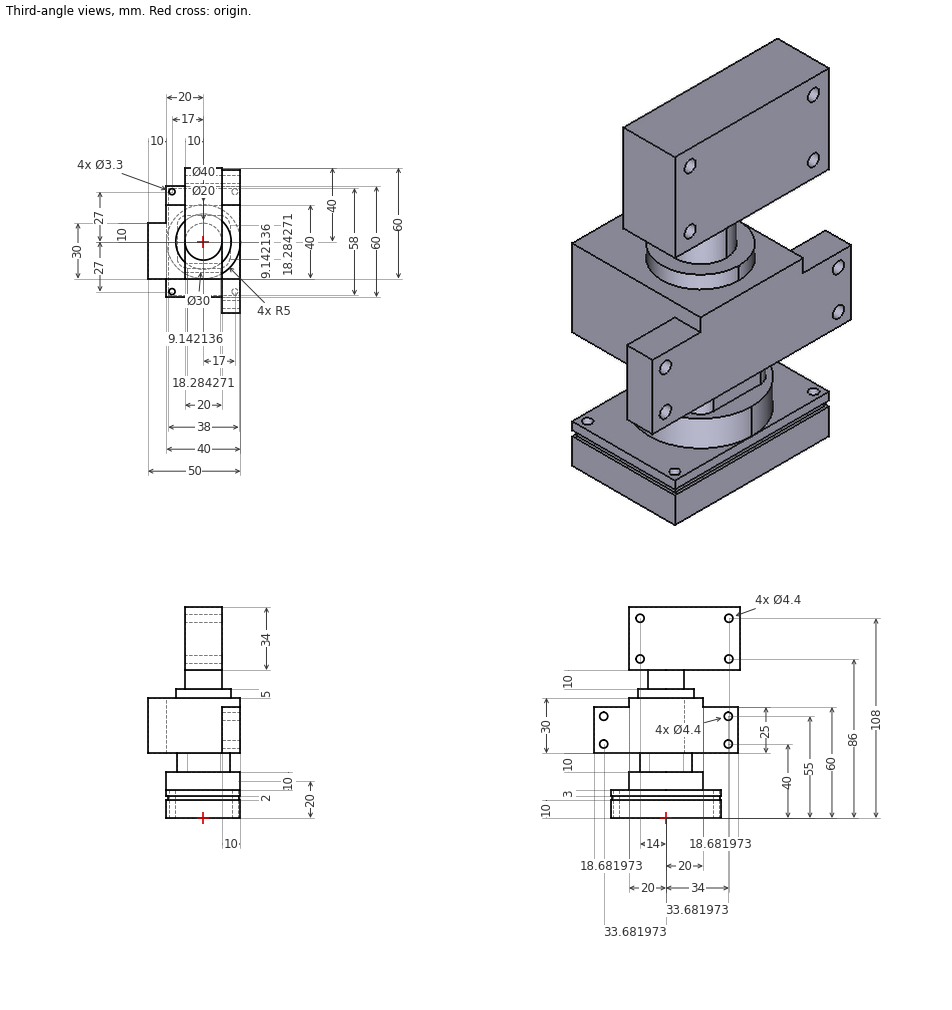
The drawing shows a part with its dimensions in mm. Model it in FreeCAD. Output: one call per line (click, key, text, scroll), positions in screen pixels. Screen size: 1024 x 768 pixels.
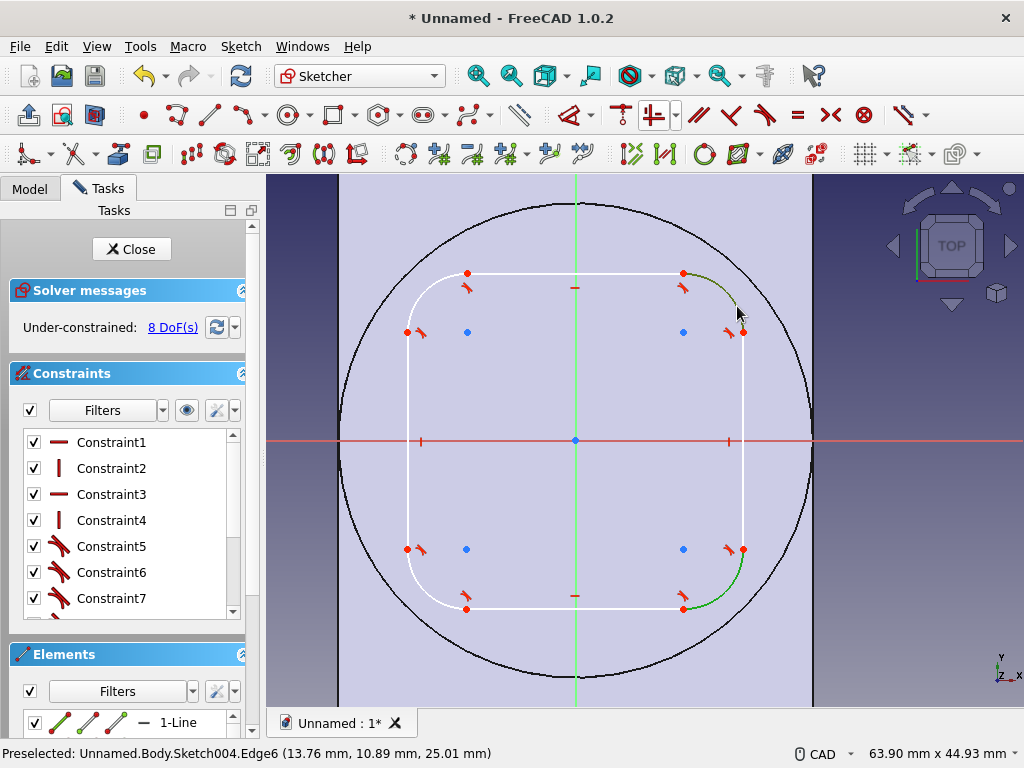
click(440, 280)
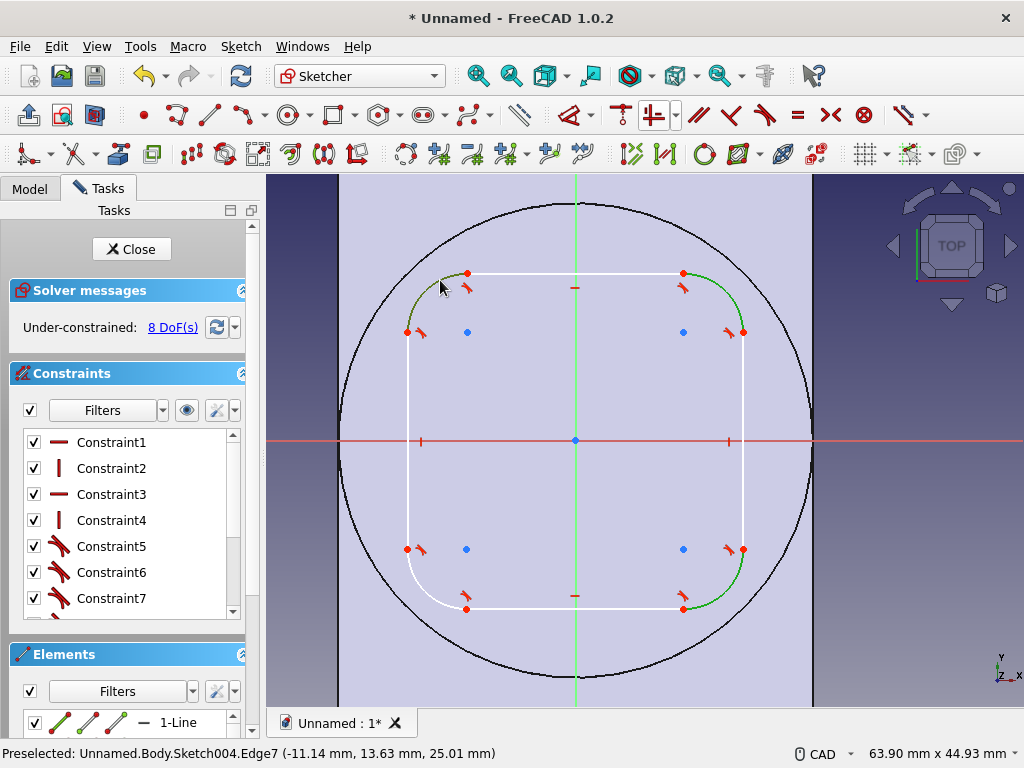
click(414, 577)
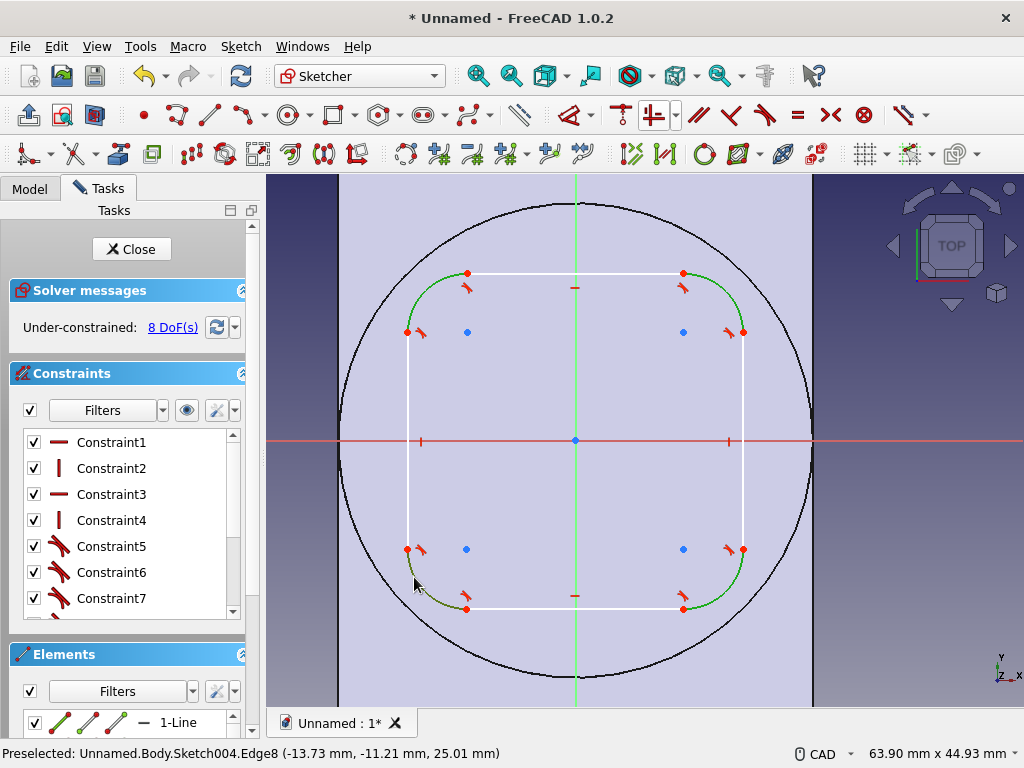
key(e)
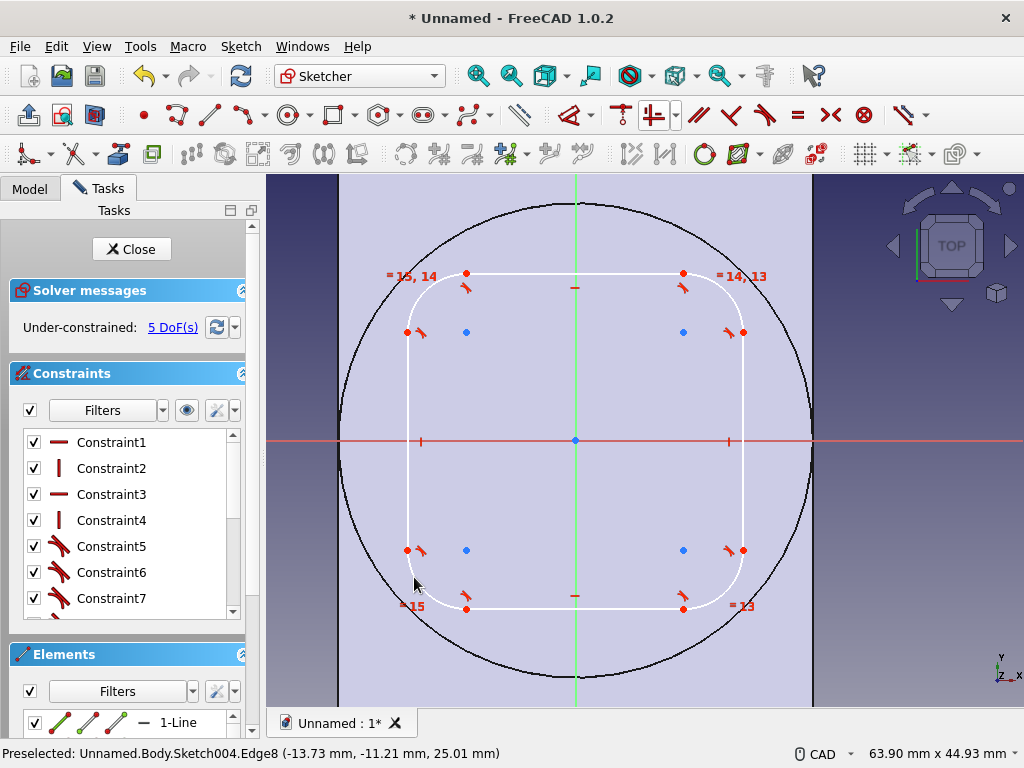
key(d)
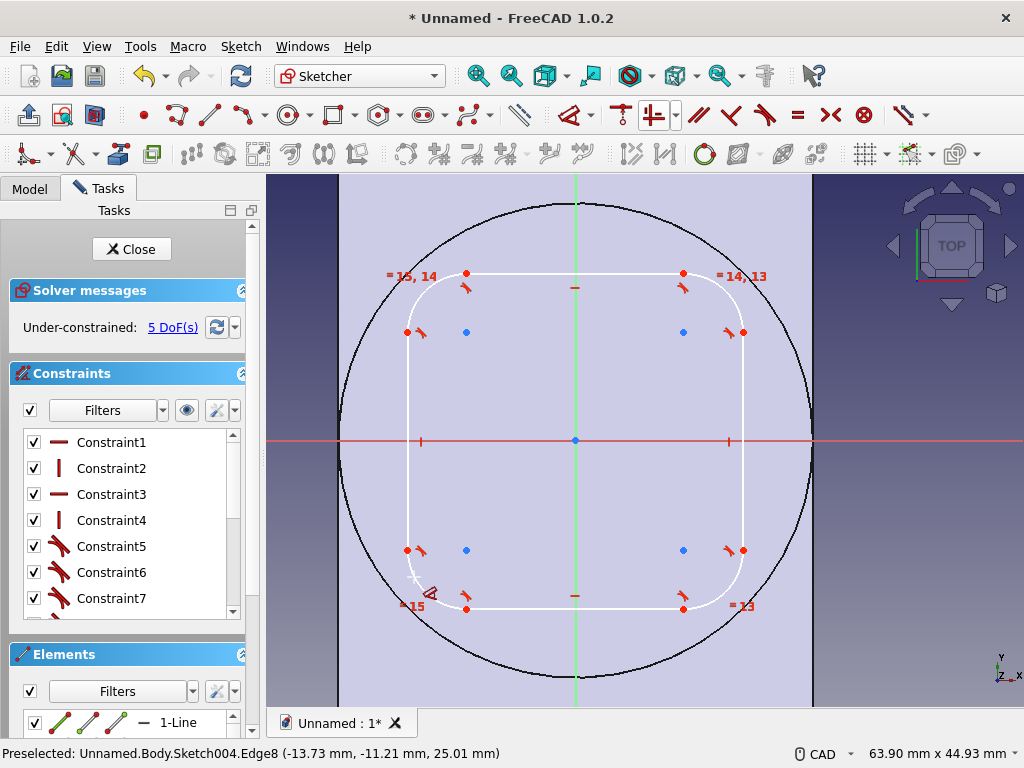
click(711, 603)
click(726, 632)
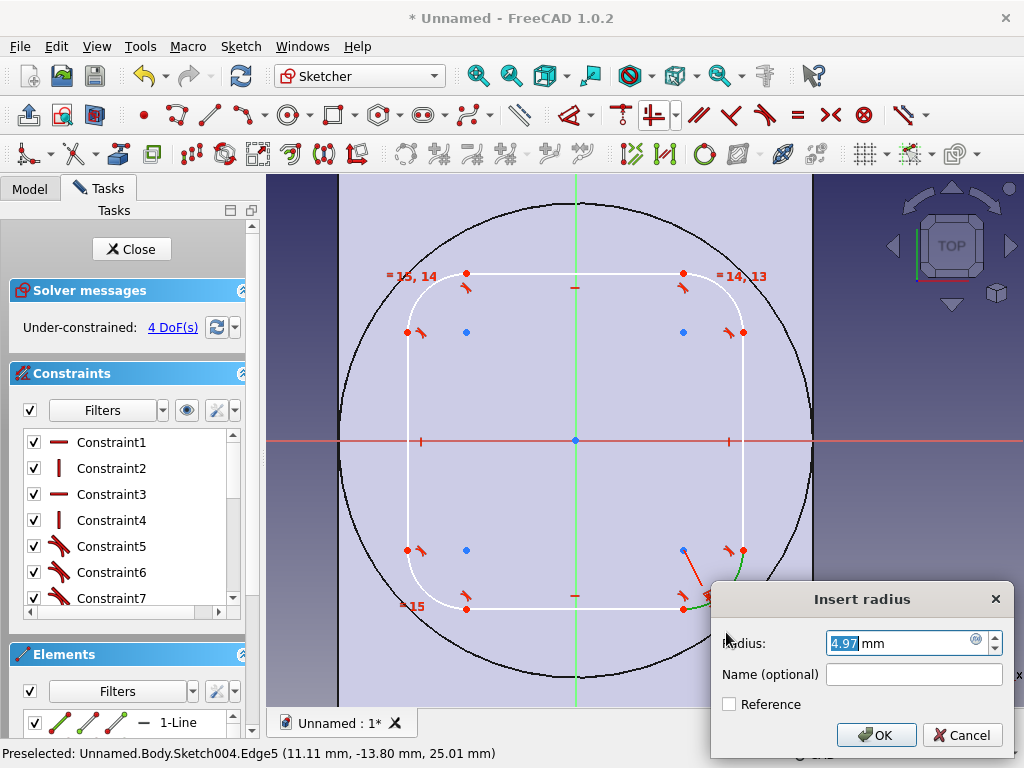
text(5)
key(Return)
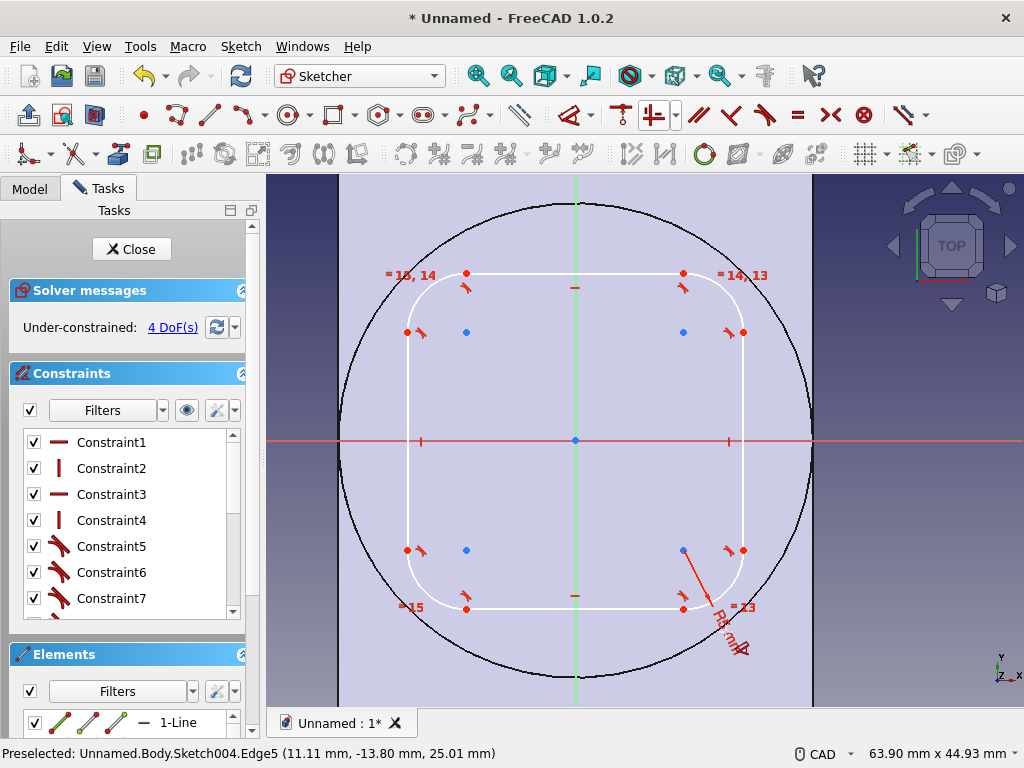
click(532, 609)
click(526, 643)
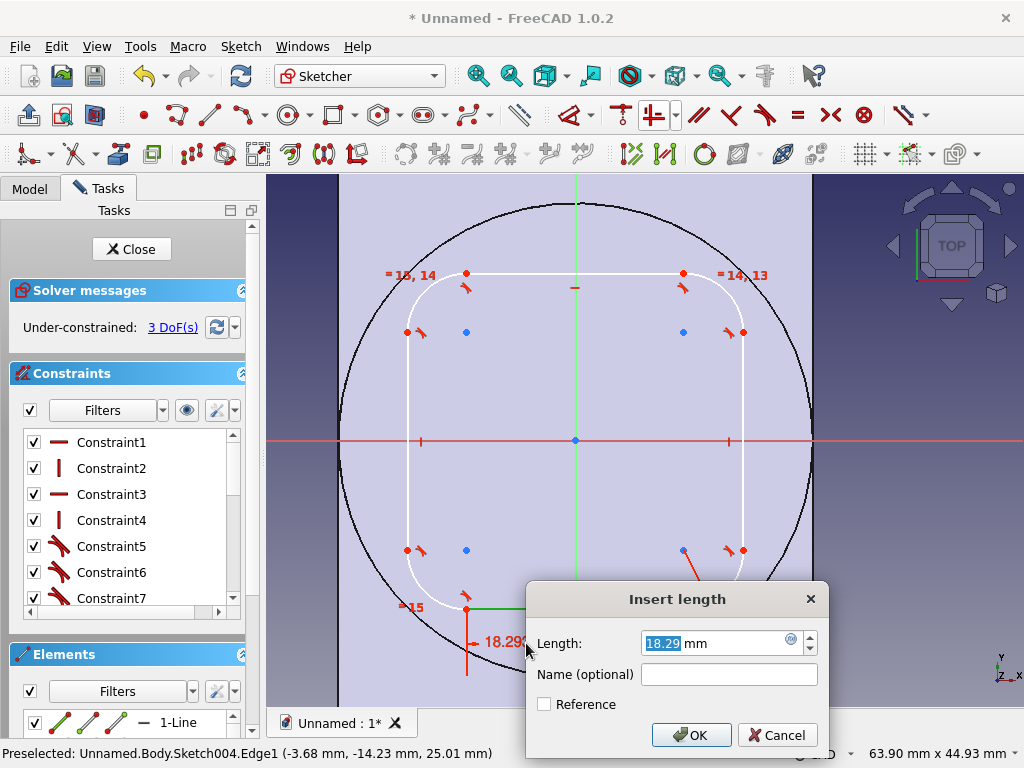
text(18.284271)
key(Return)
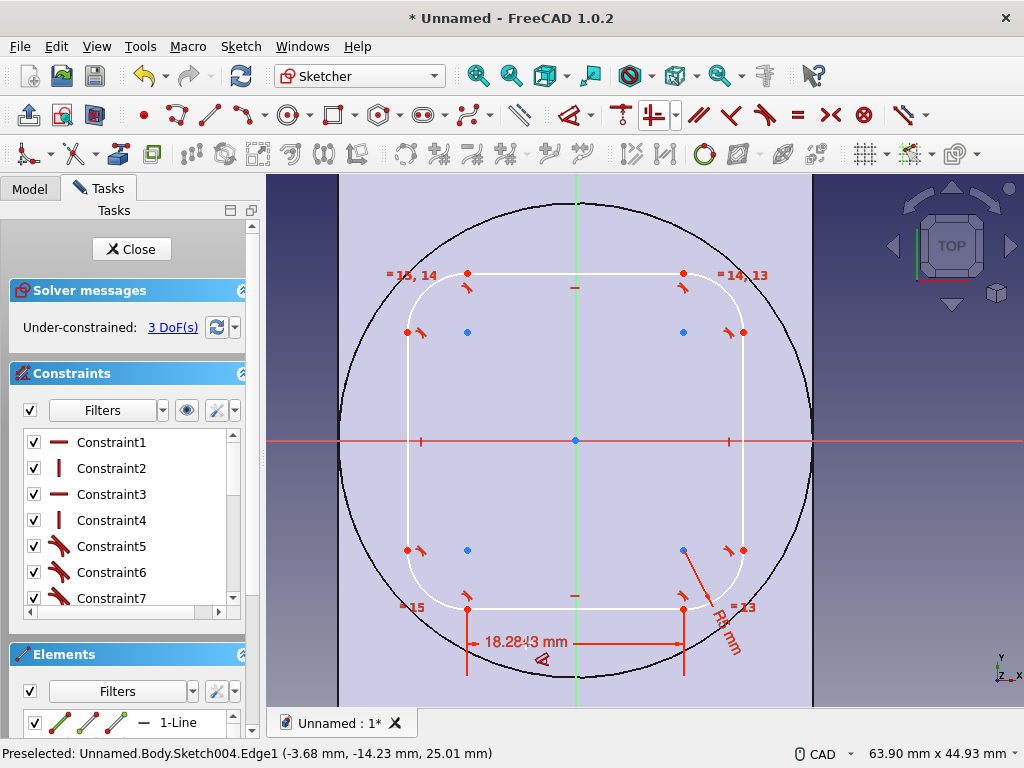
click(743, 485)
click(777, 392)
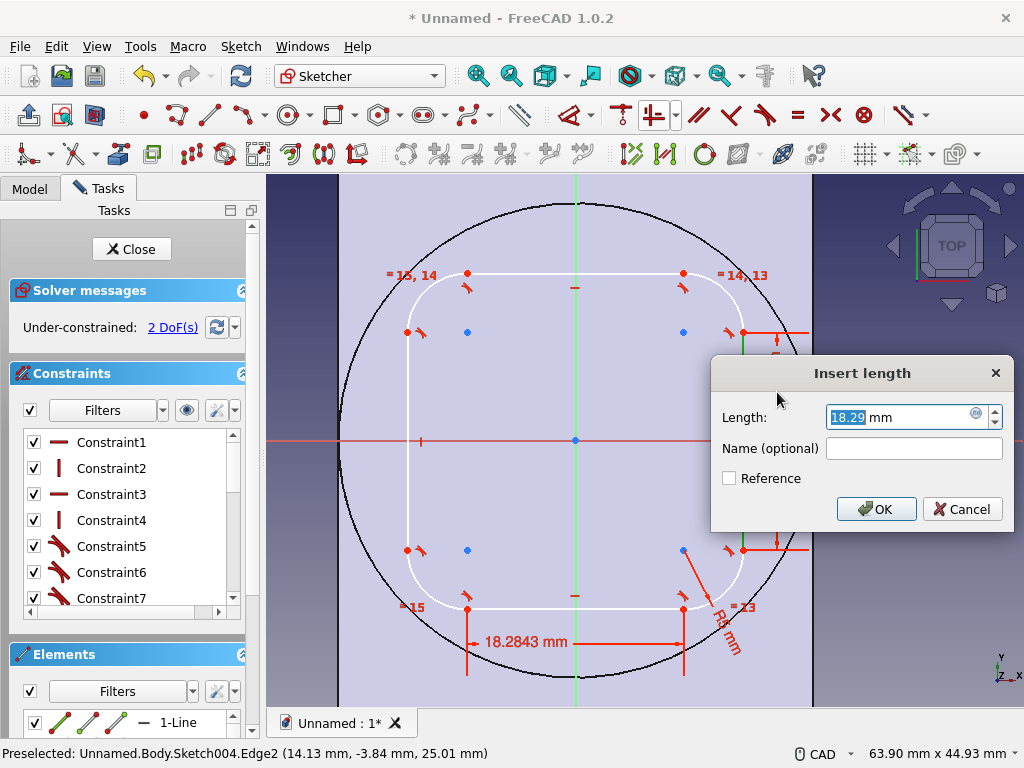
text(18.284271)
key(Return)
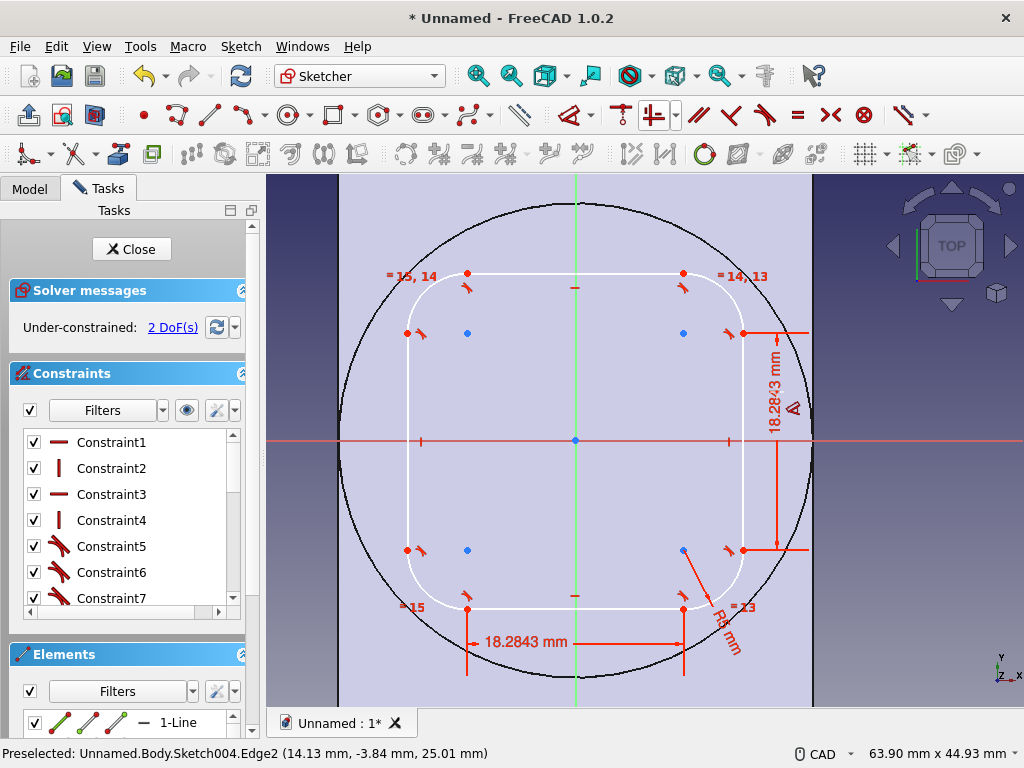
click(467, 609)
click(521, 406)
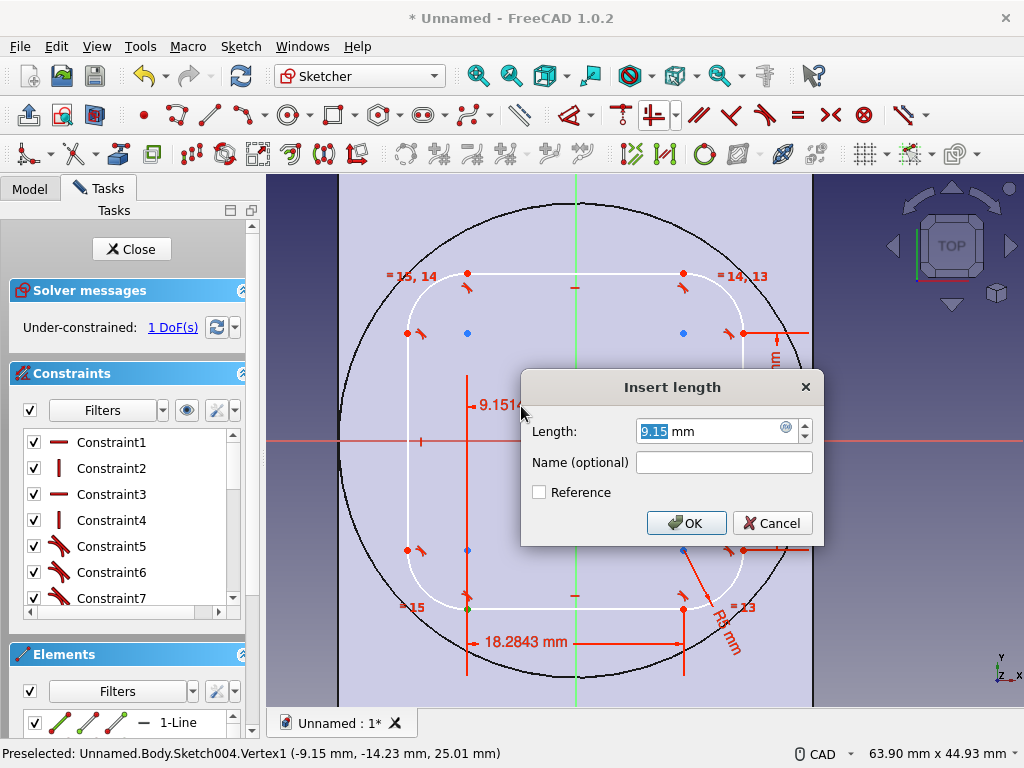
text(9.142136)
key(Return)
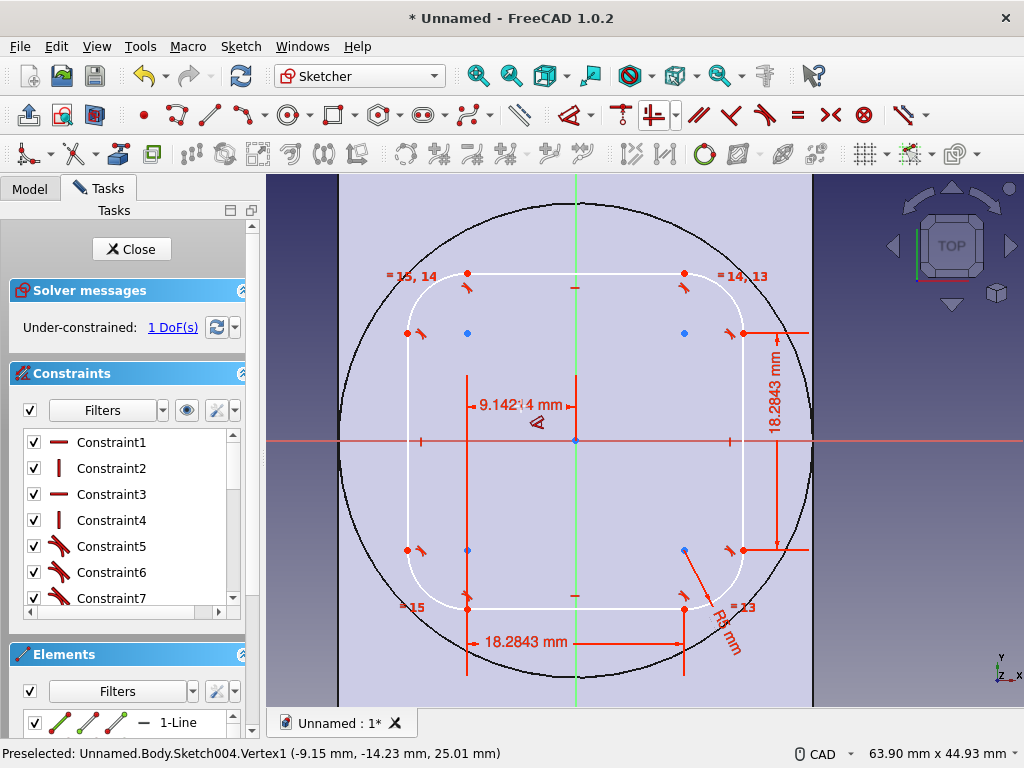
click(743, 550)
click(777, 495)